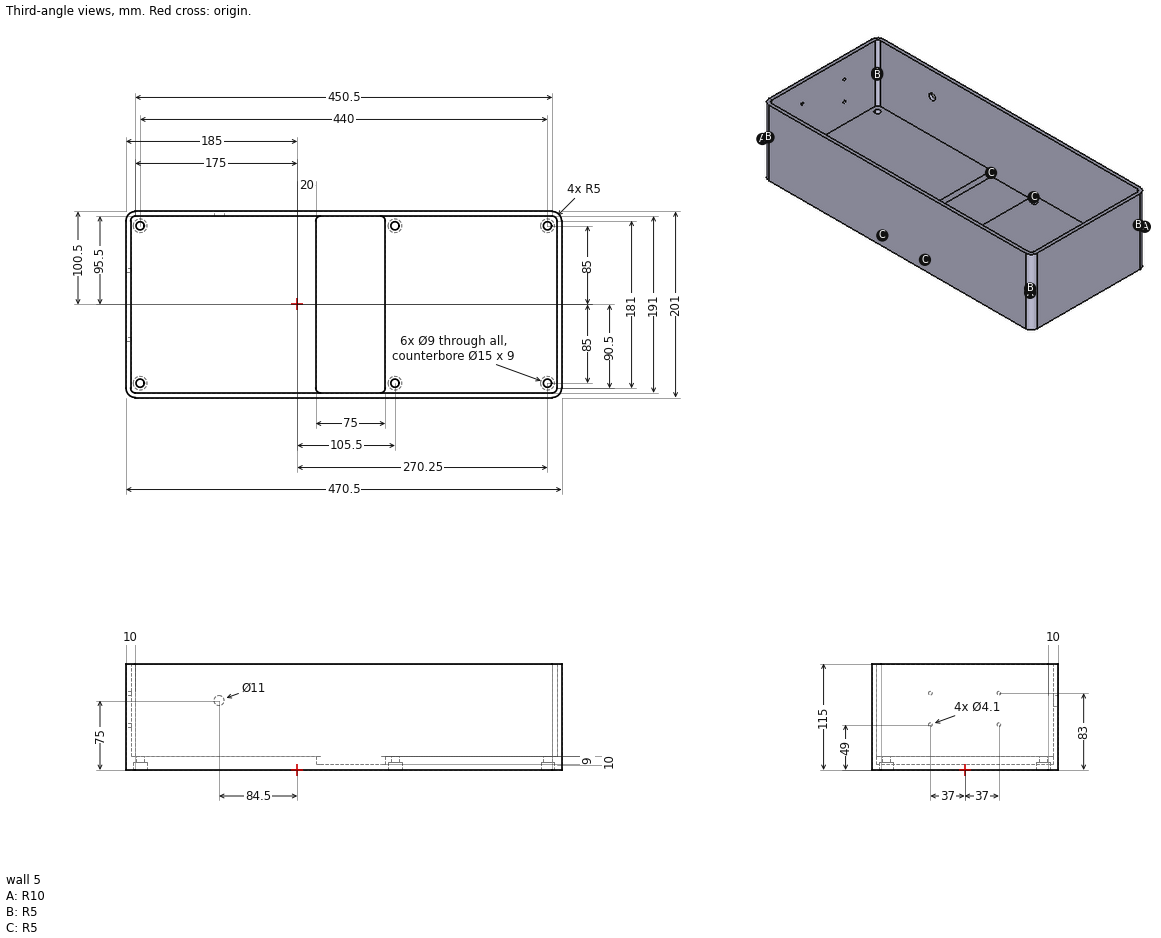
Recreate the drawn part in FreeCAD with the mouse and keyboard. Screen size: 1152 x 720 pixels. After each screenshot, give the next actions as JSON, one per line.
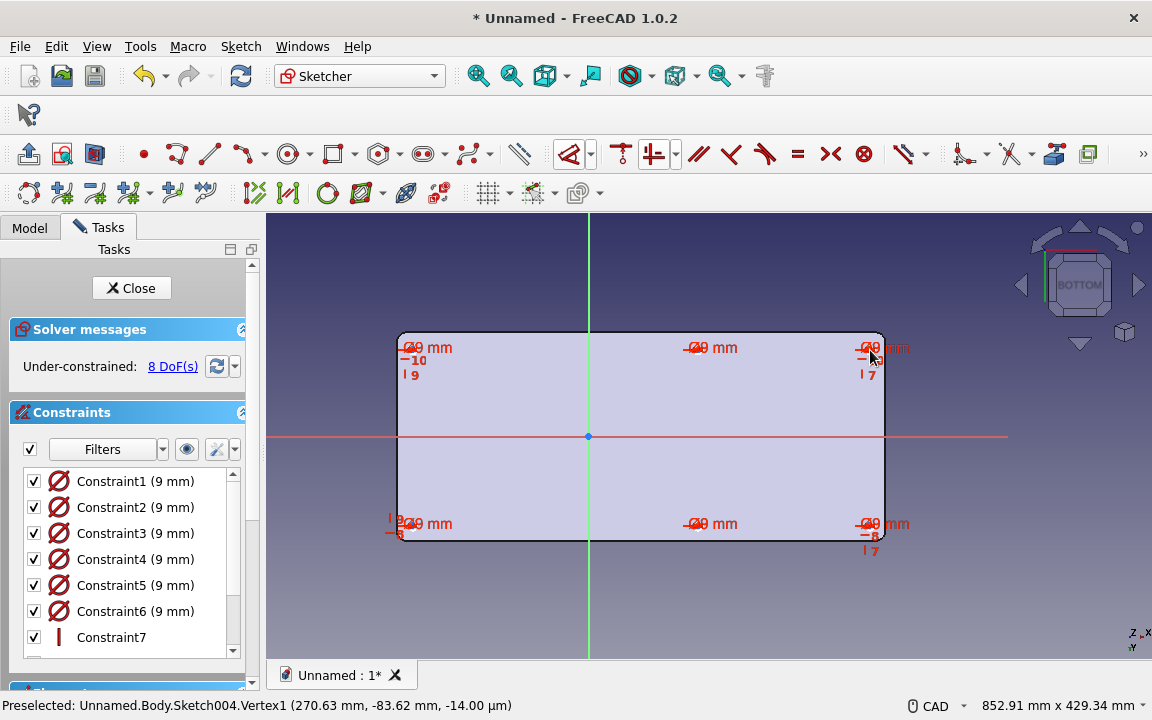
{"action": "left_click", "coordinate": [698, 350]}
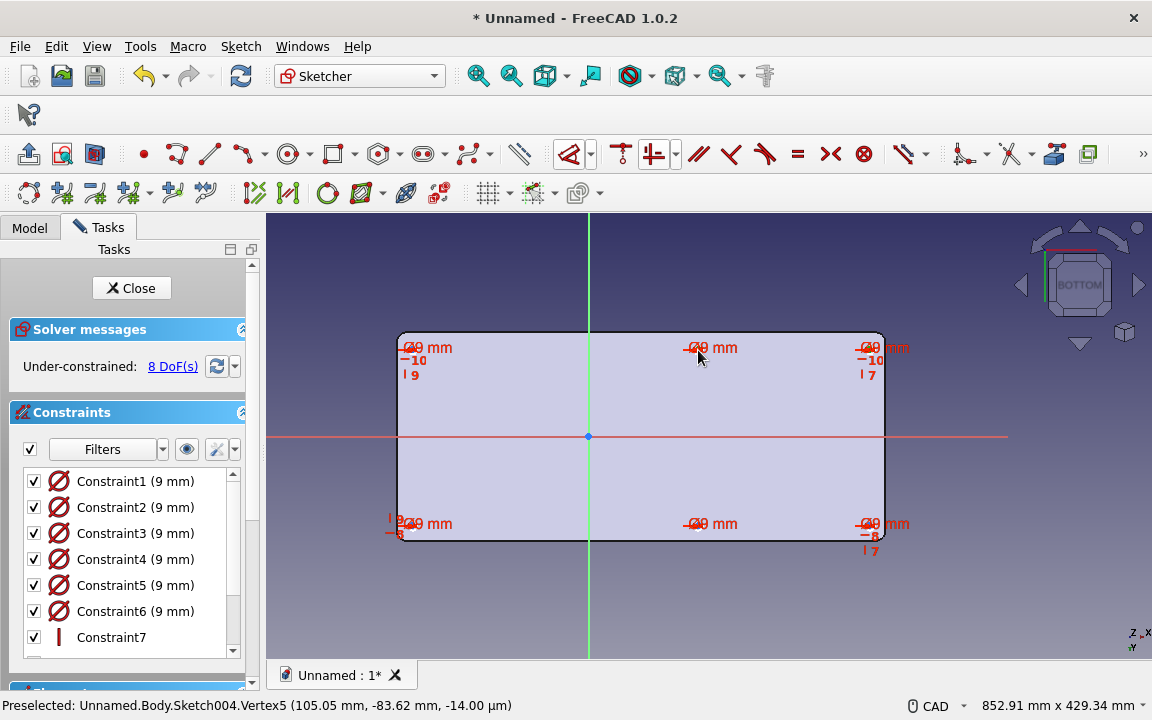
{"action": "key", "text": "h"}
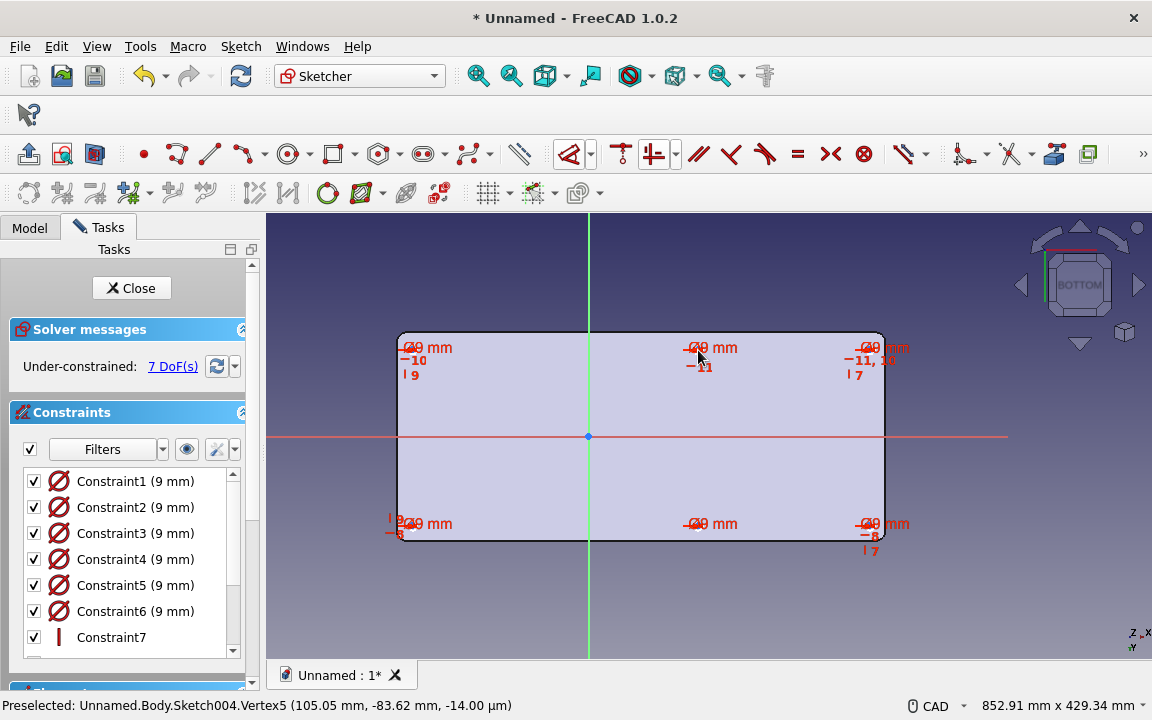
{"action": "left_click", "coordinate": [698, 350]}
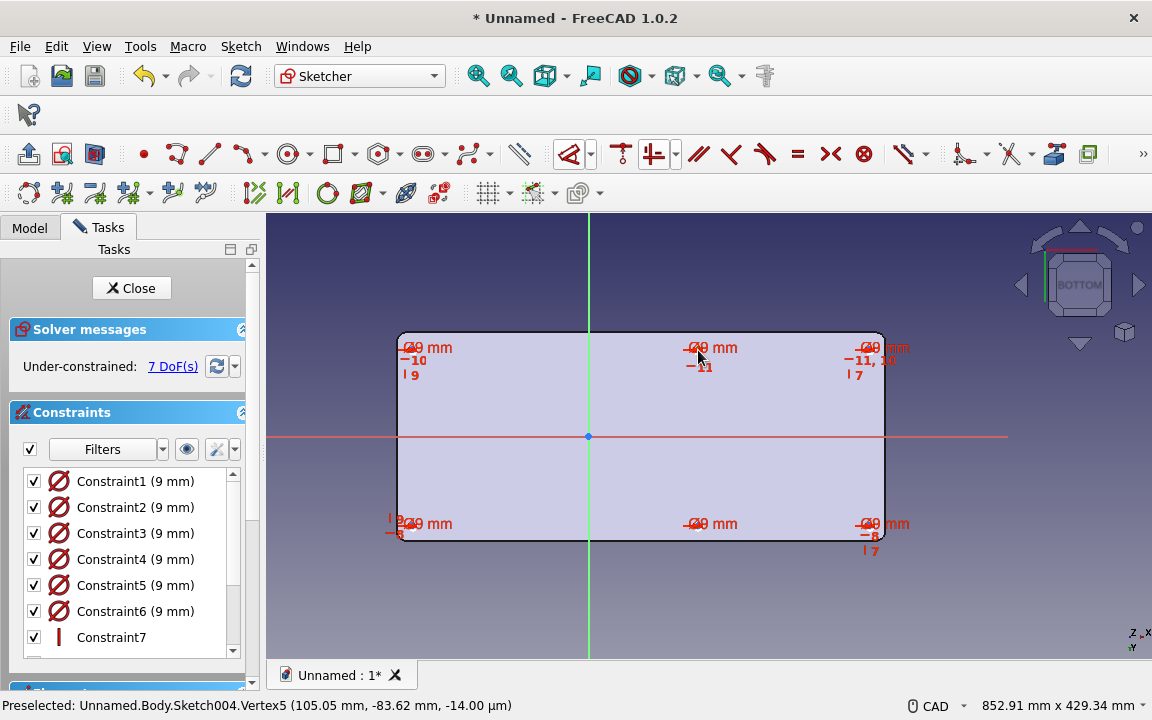
{"action": "left_click", "coordinate": [698, 526]}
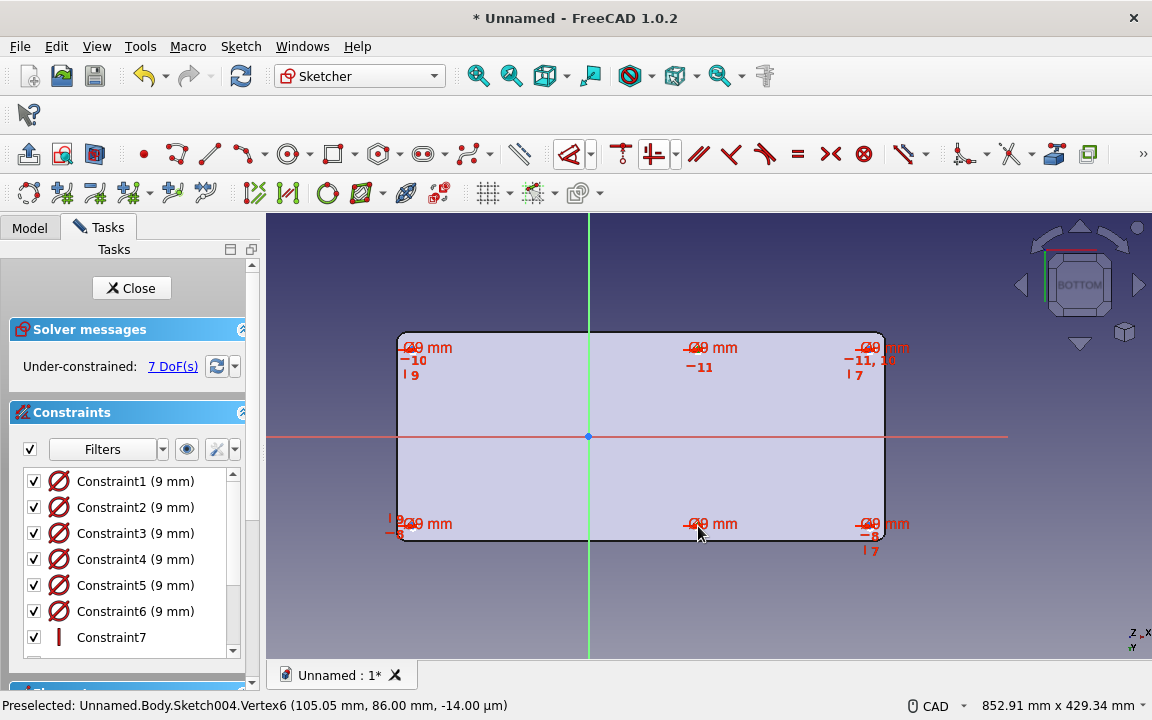
{"action": "key", "text": "v"}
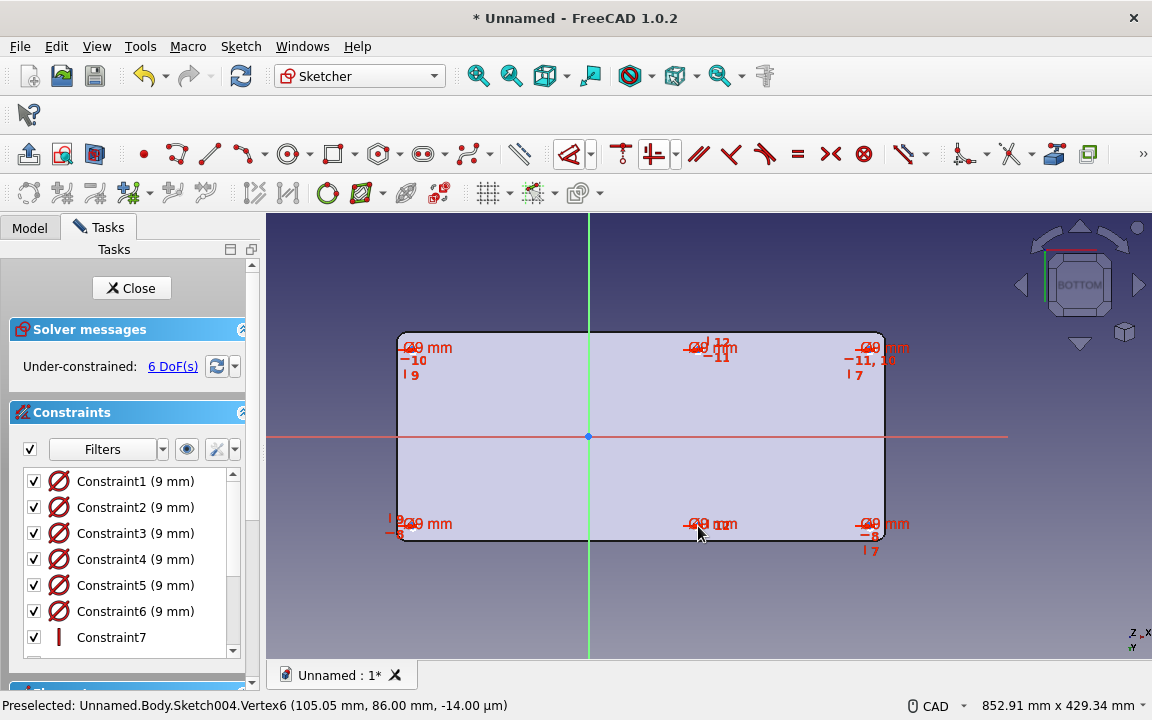
{"action": "left_click", "coordinate": [870, 526]}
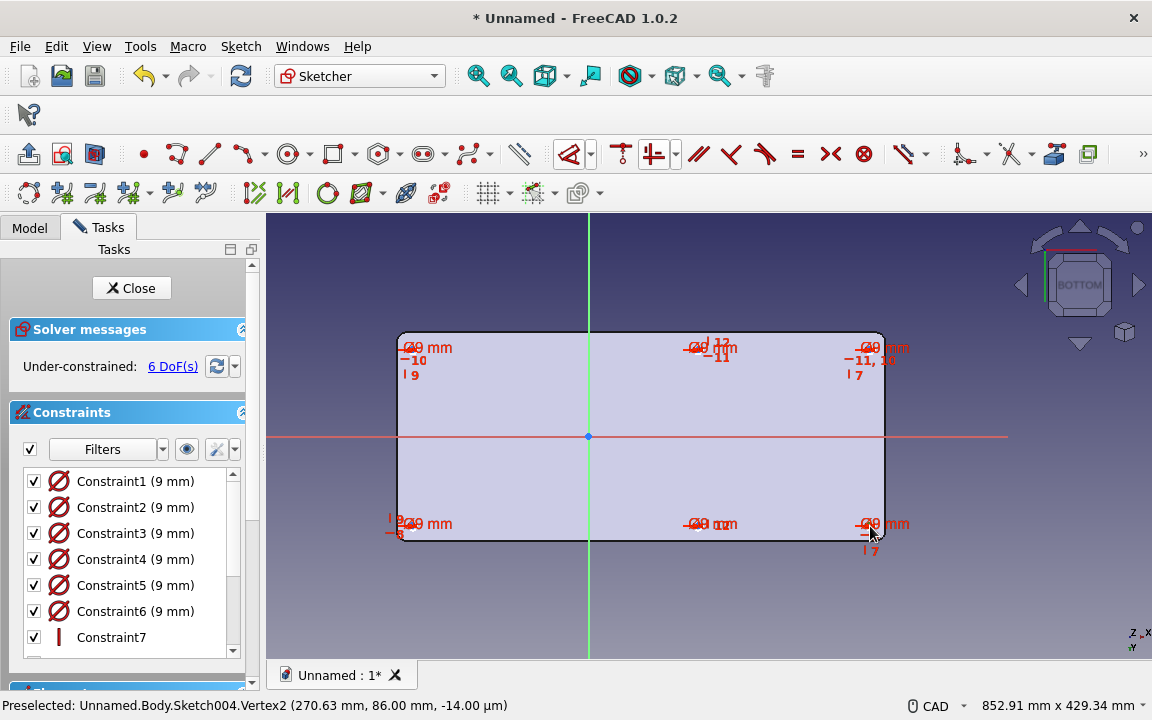
{"action": "left_click", "coordinate": [698, 526]}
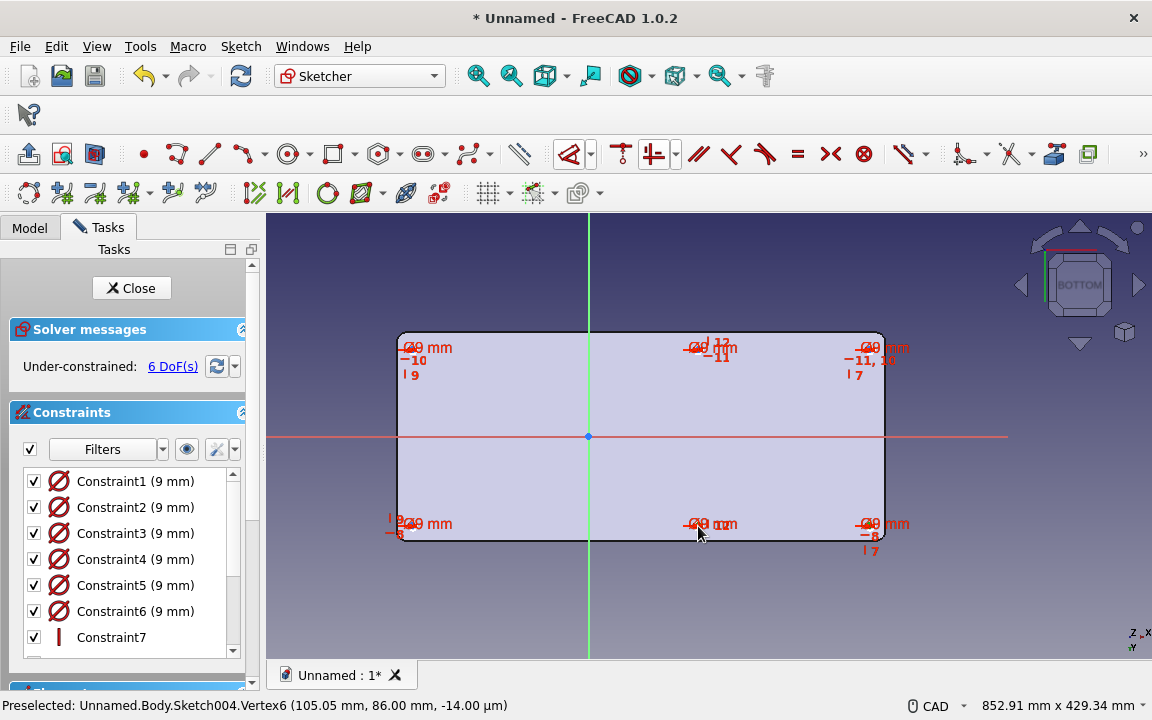
{"action": "key", "text": "h"}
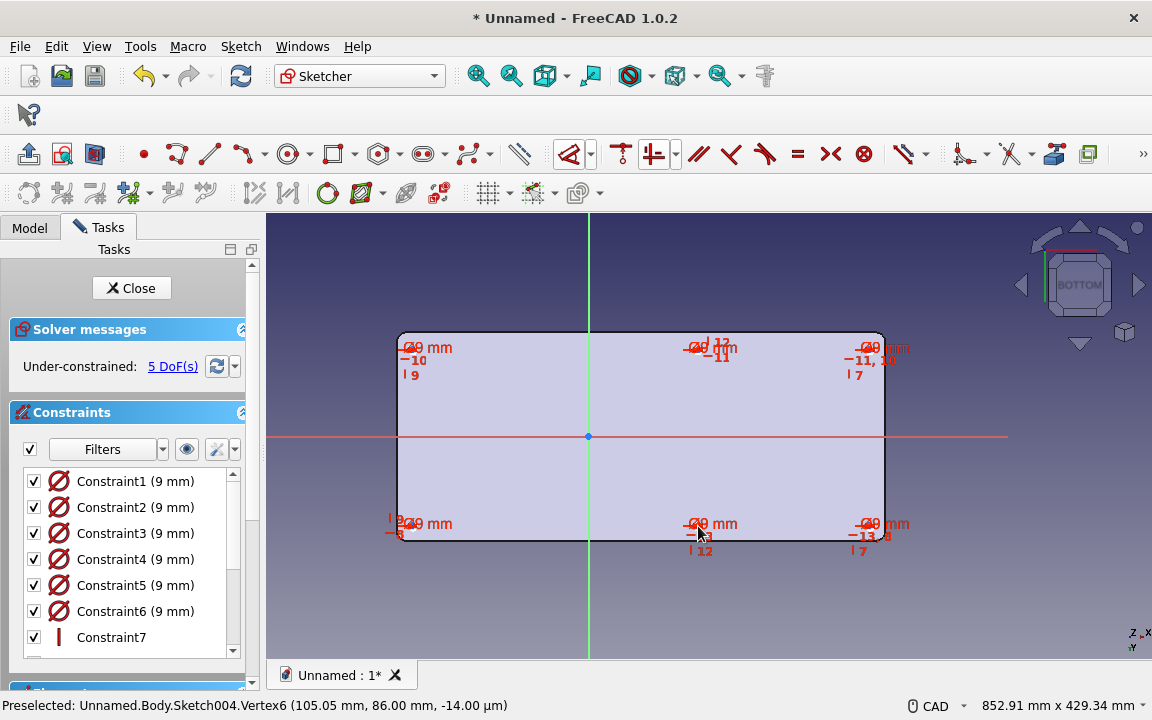
{"action": "key", "text": "d"}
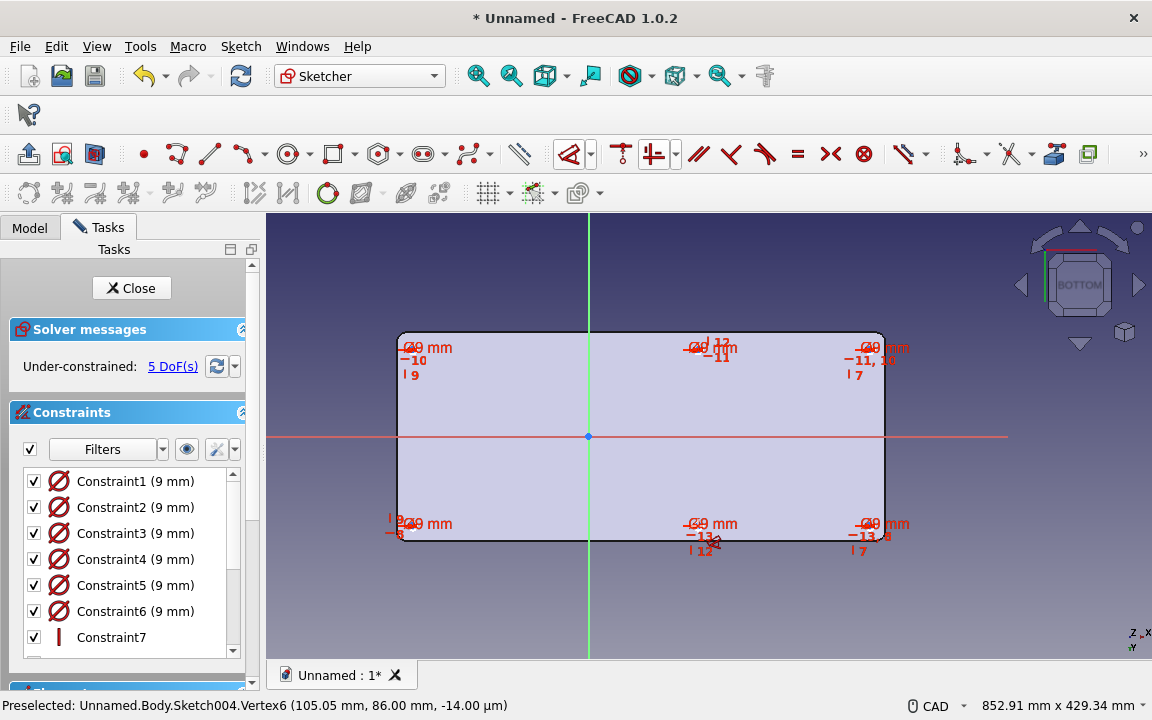
{"action": "left_click", "coordinate": [870, 350]}
{"action": "left_click", "coordinate": [904, 393]}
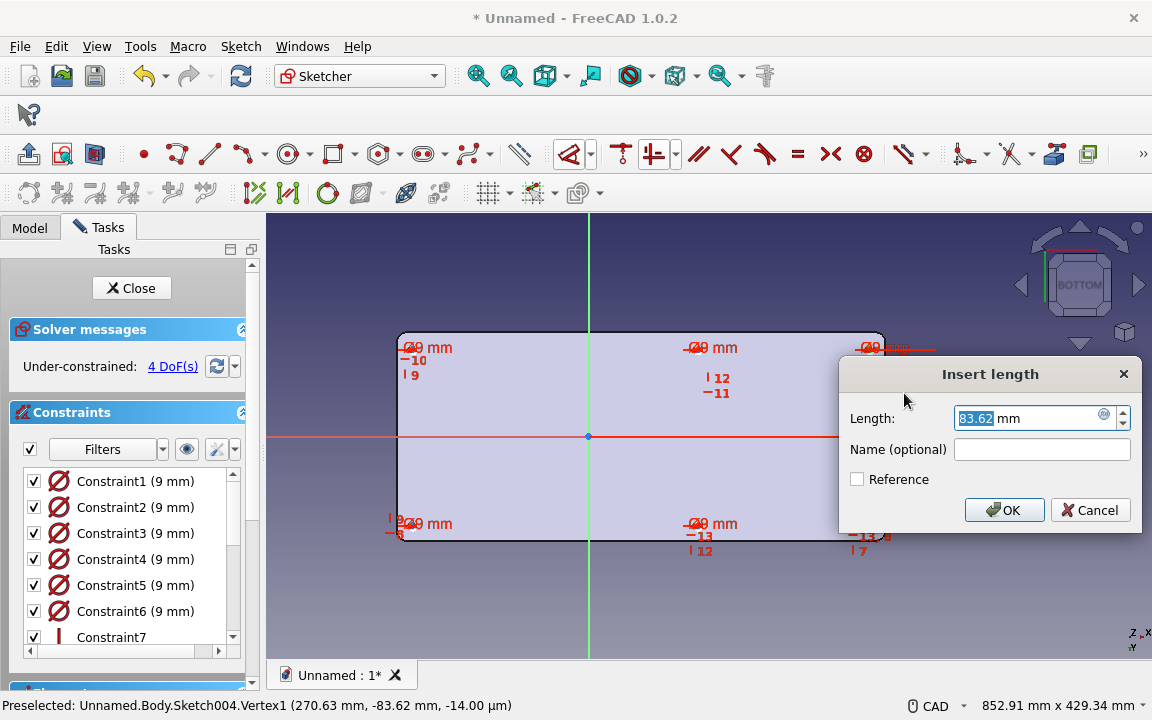
{"action": "type", "text": "85"}
{"action": "key", "text": "Return"}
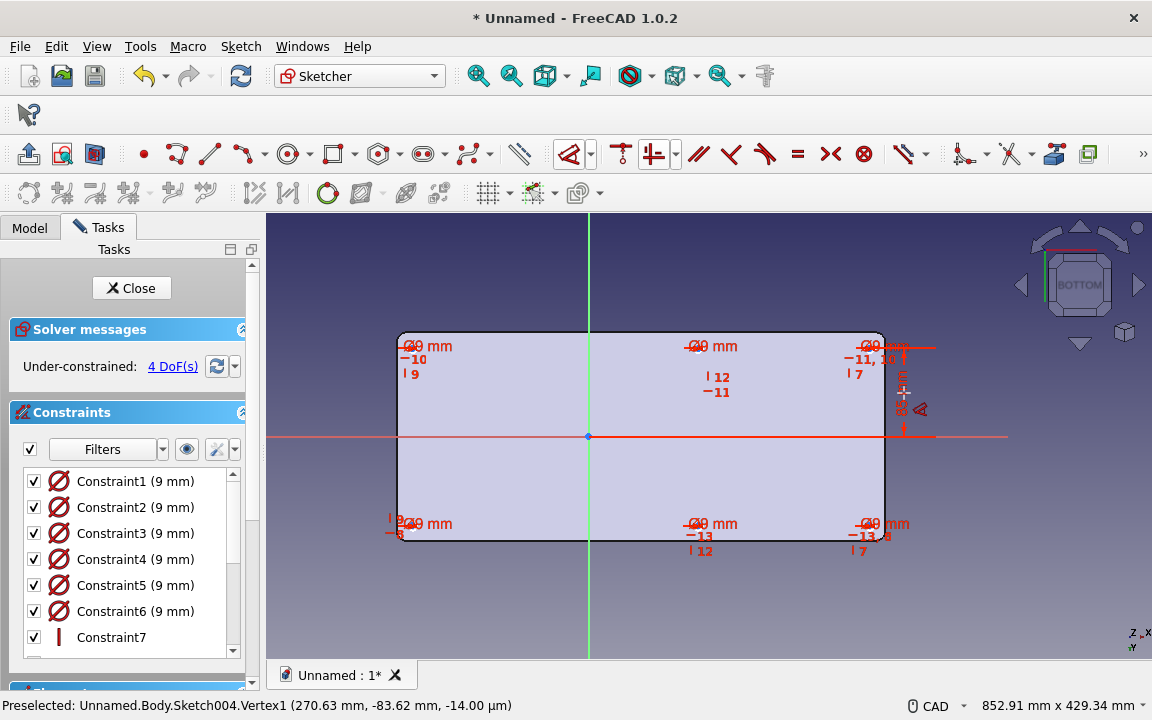
{"action": "left_click", "coordinate": [870, 526]}
{"action": "left_click", "coordinate": [904, 481]}